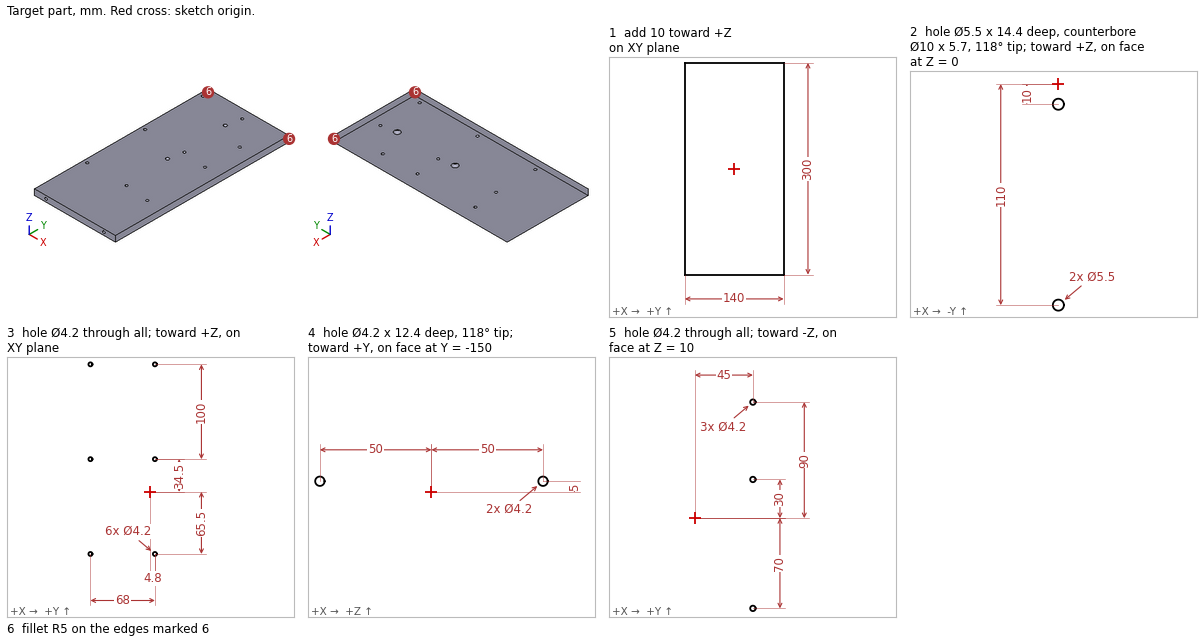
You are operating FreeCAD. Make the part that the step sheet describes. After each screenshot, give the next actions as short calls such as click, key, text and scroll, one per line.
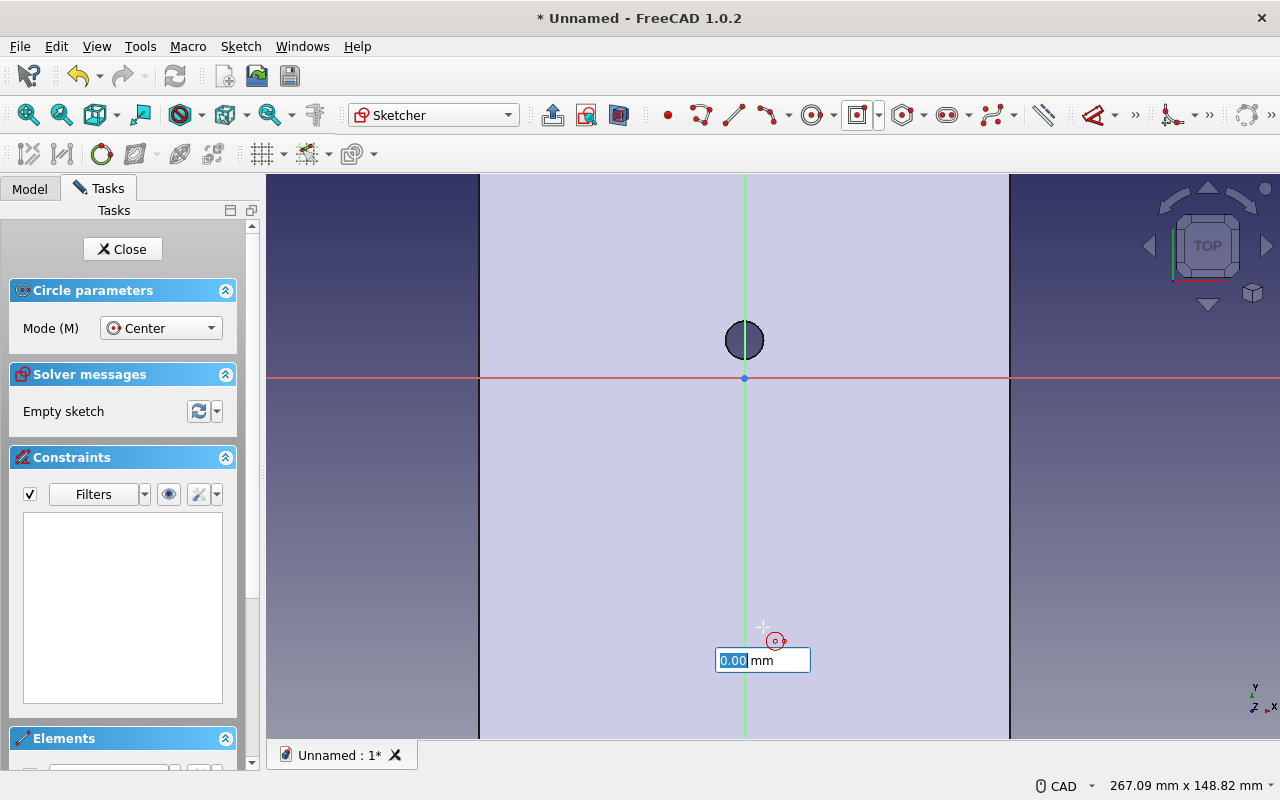
scroll(768, 621, up, 4)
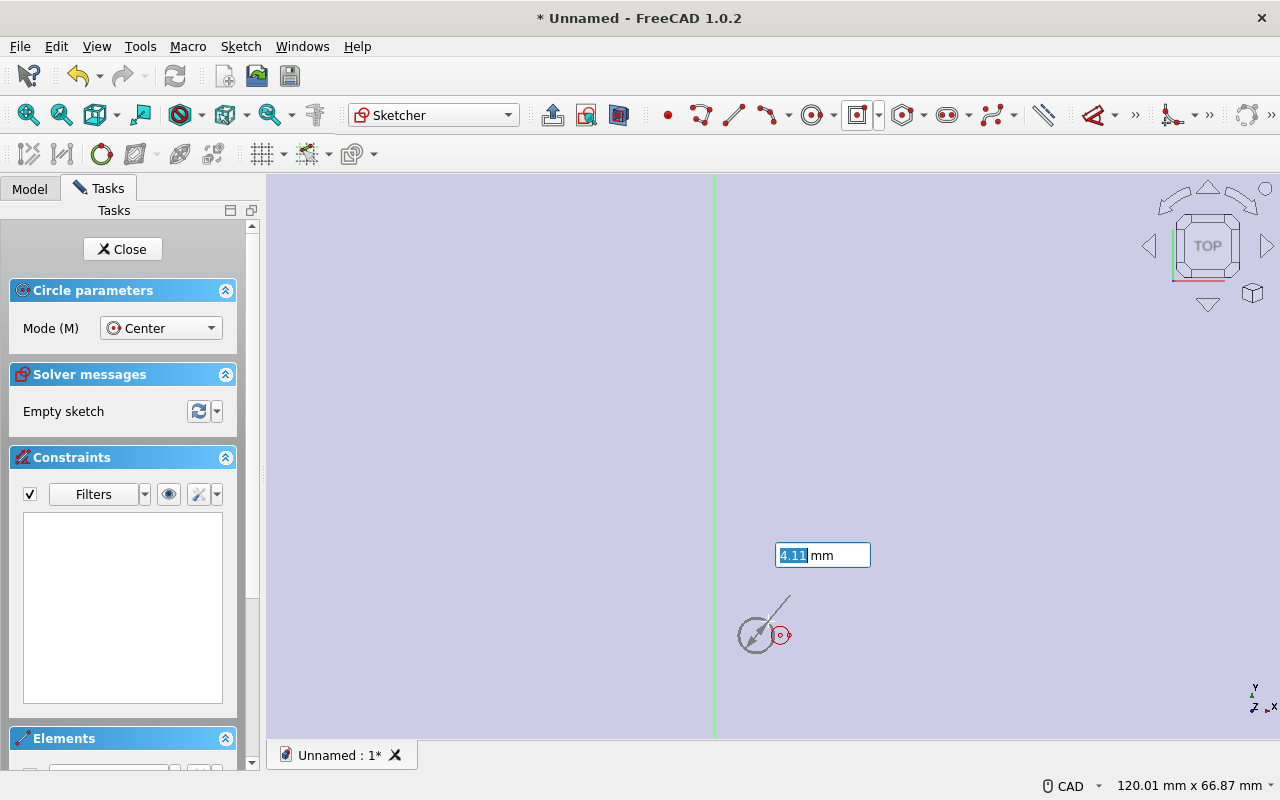
click(768, 621)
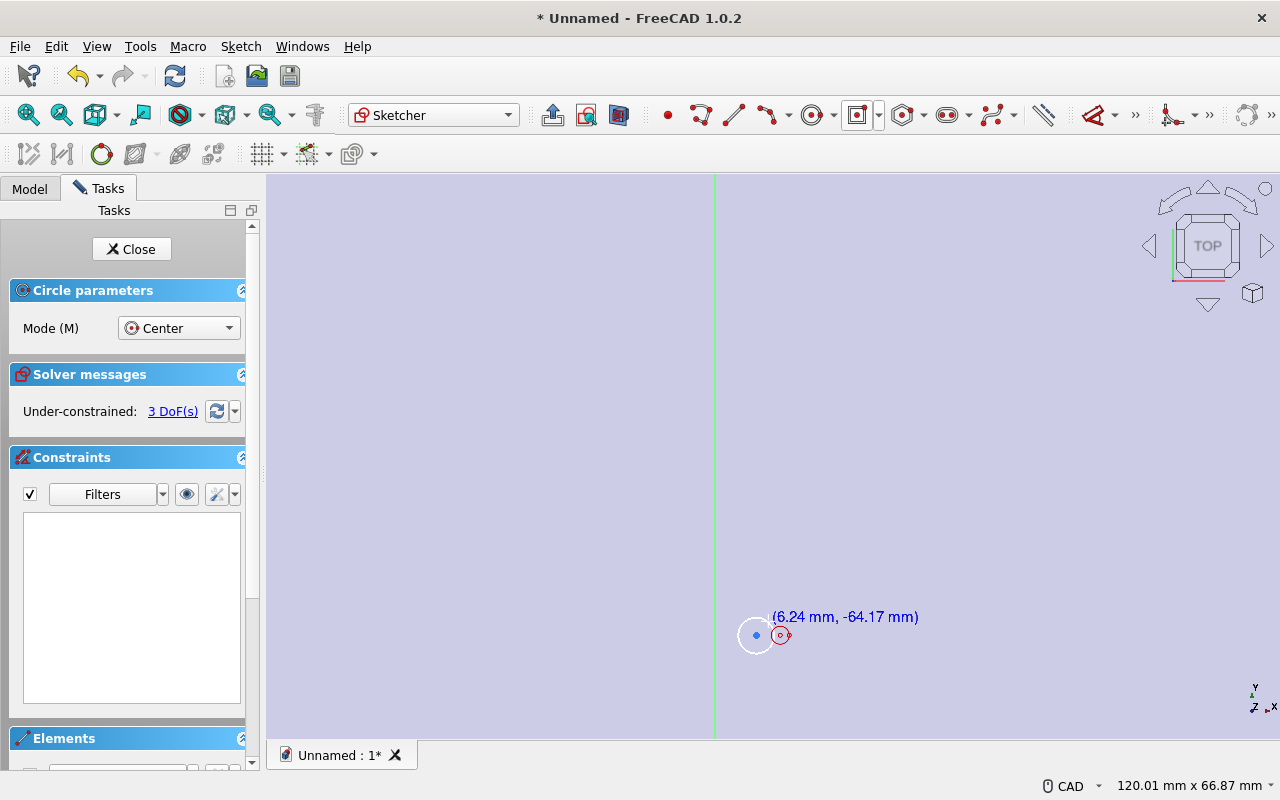
scroll(764, 626, down, 8)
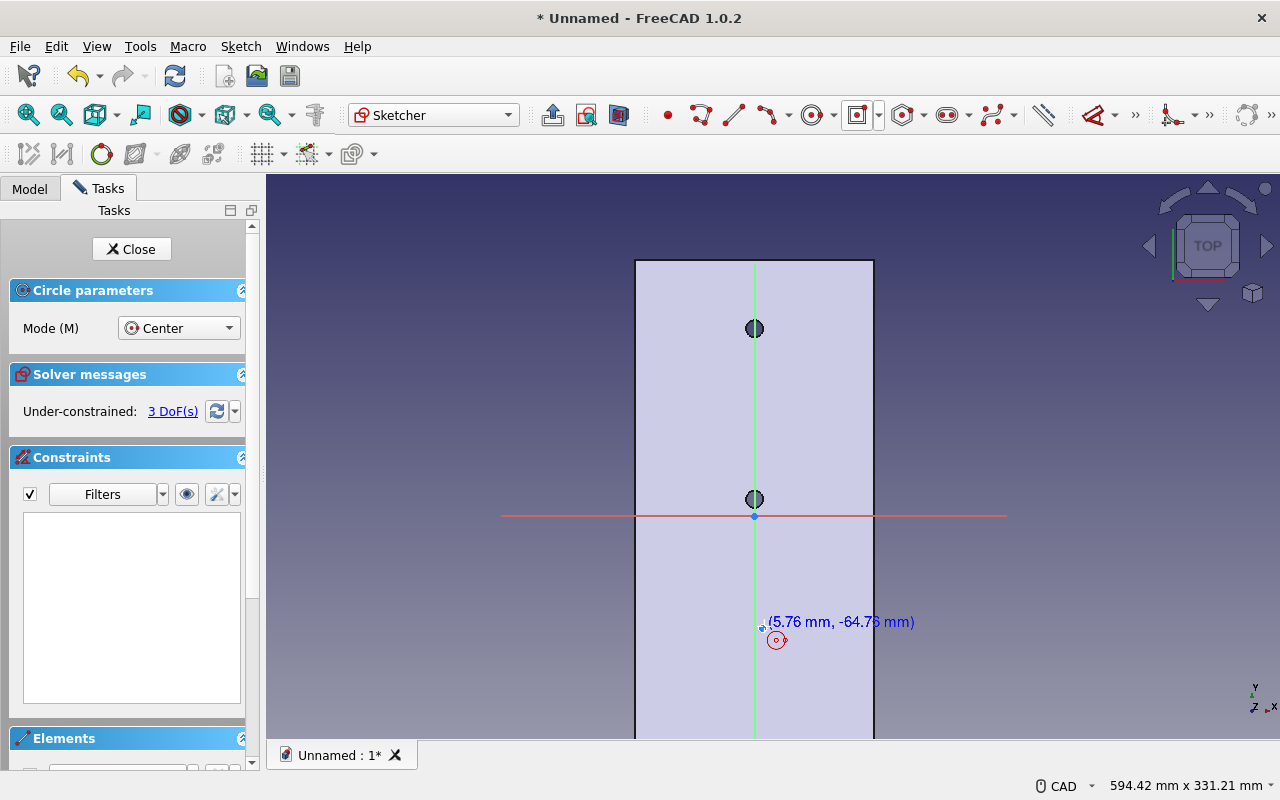
scroll(647, 628, up, 10)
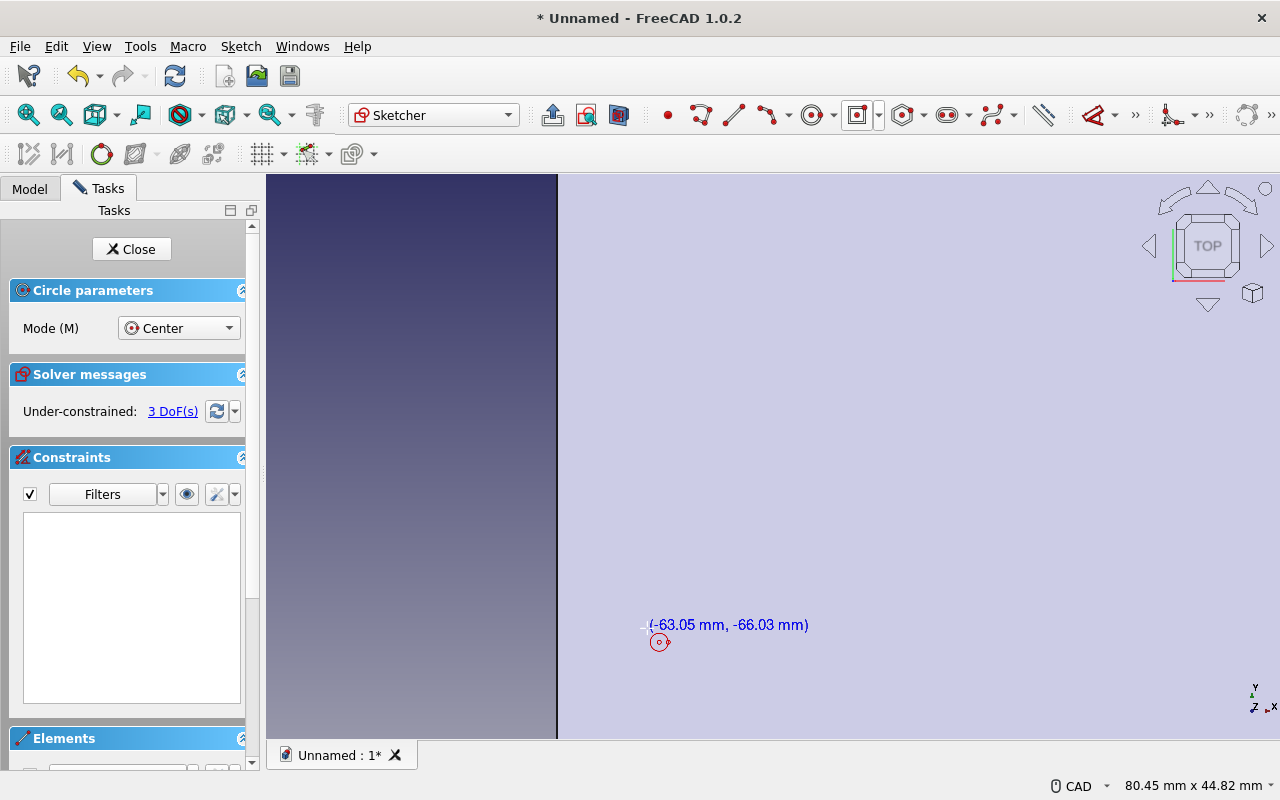
scroll(647, 628, down, 10)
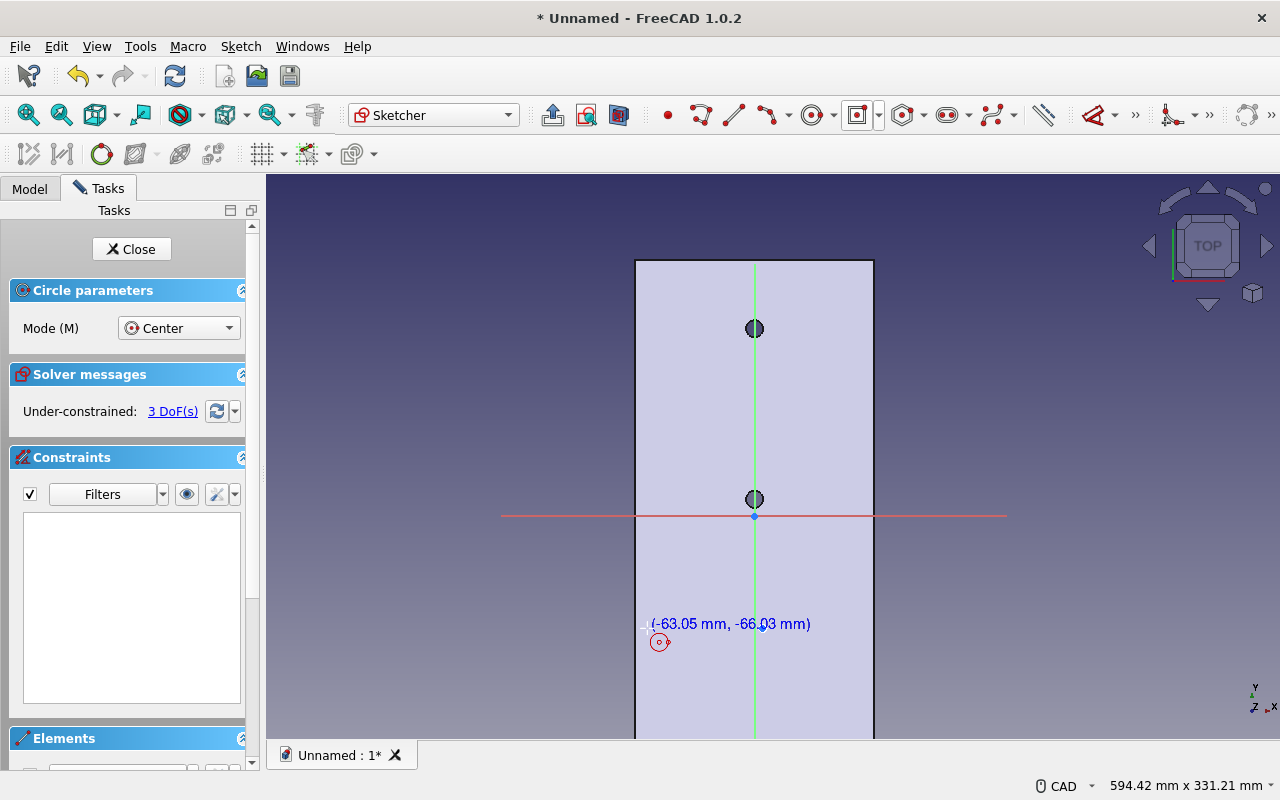
click(647, 628)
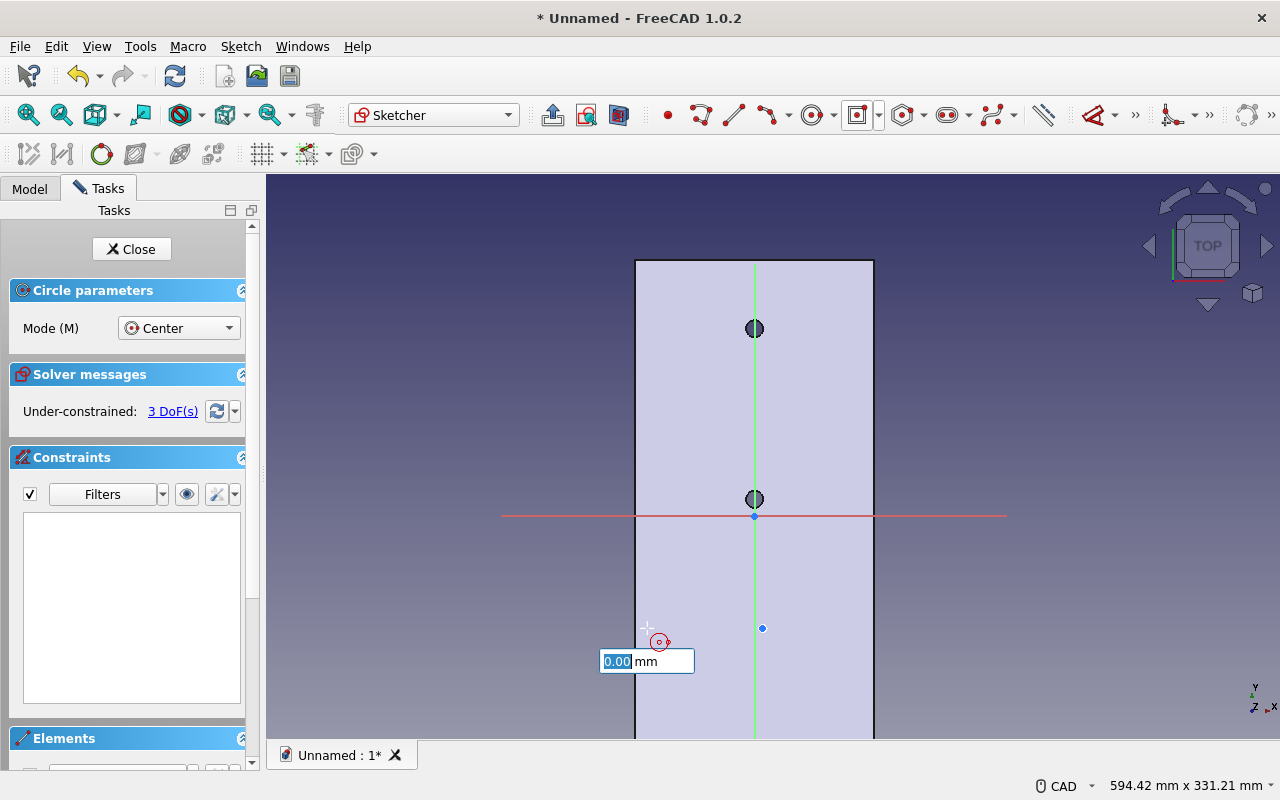
scroll(649, 626, up, 8)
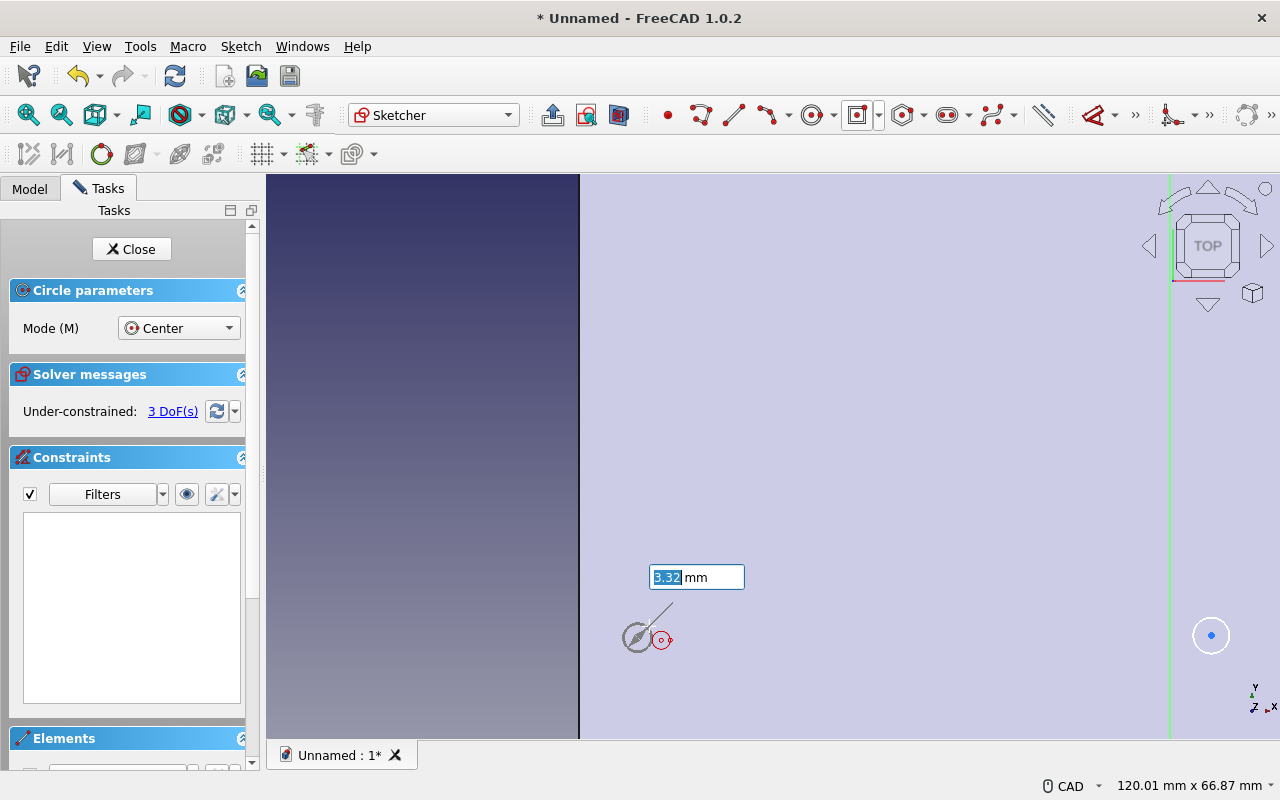
click(649, 621)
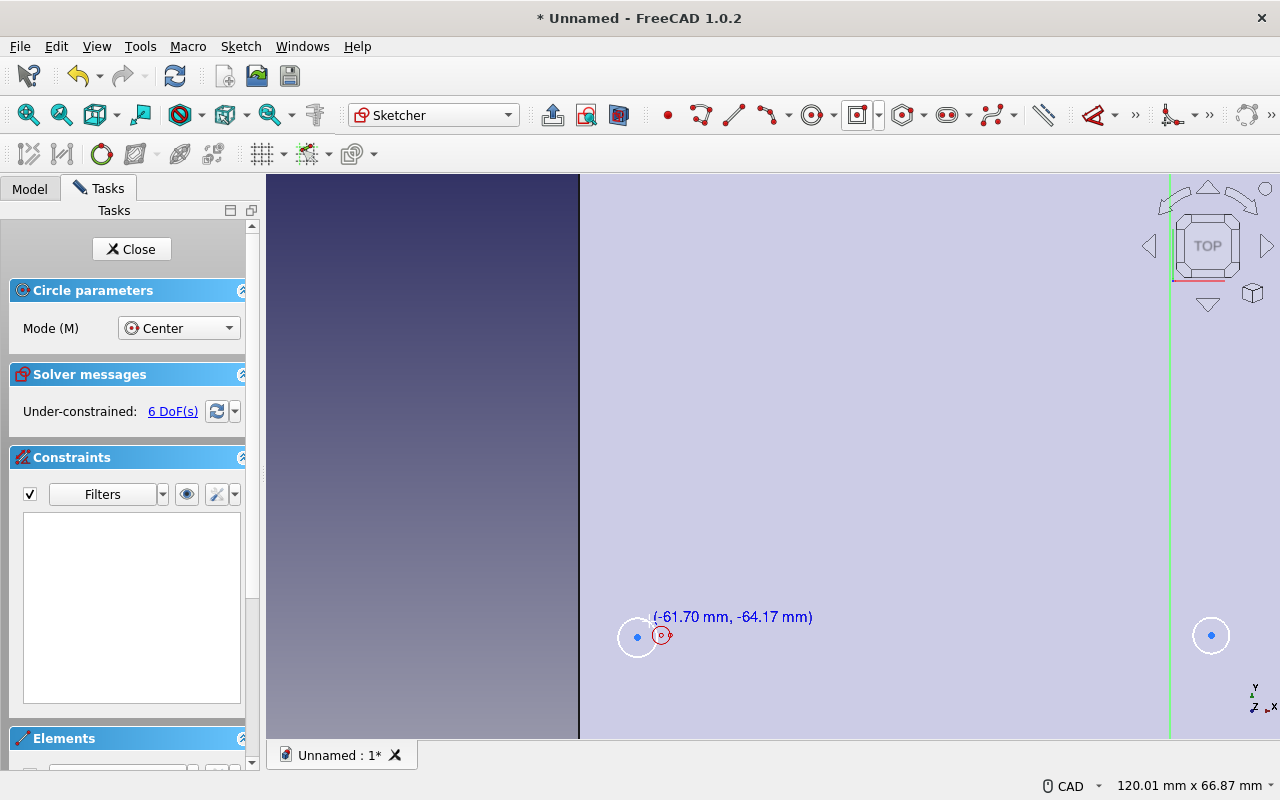
scroll(649, 626, down, 8)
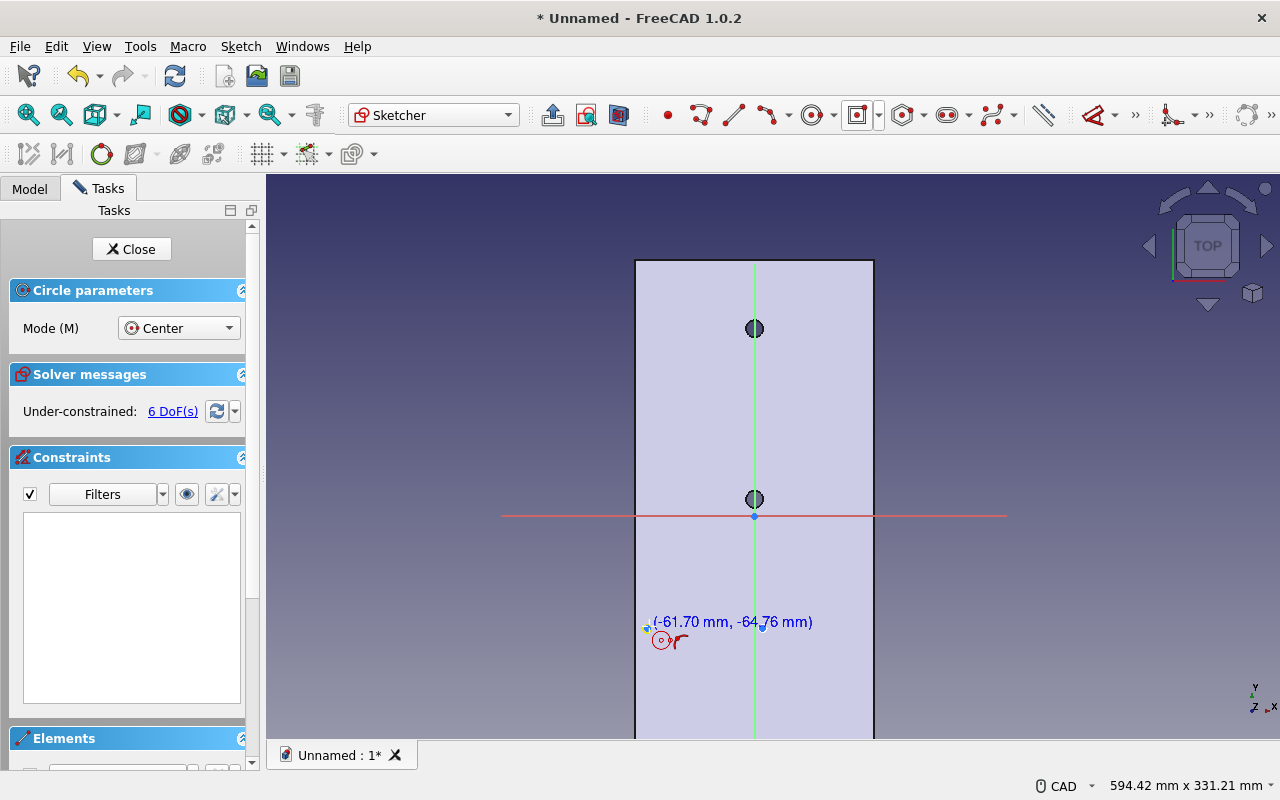
scroll(763, 458, up, 10)